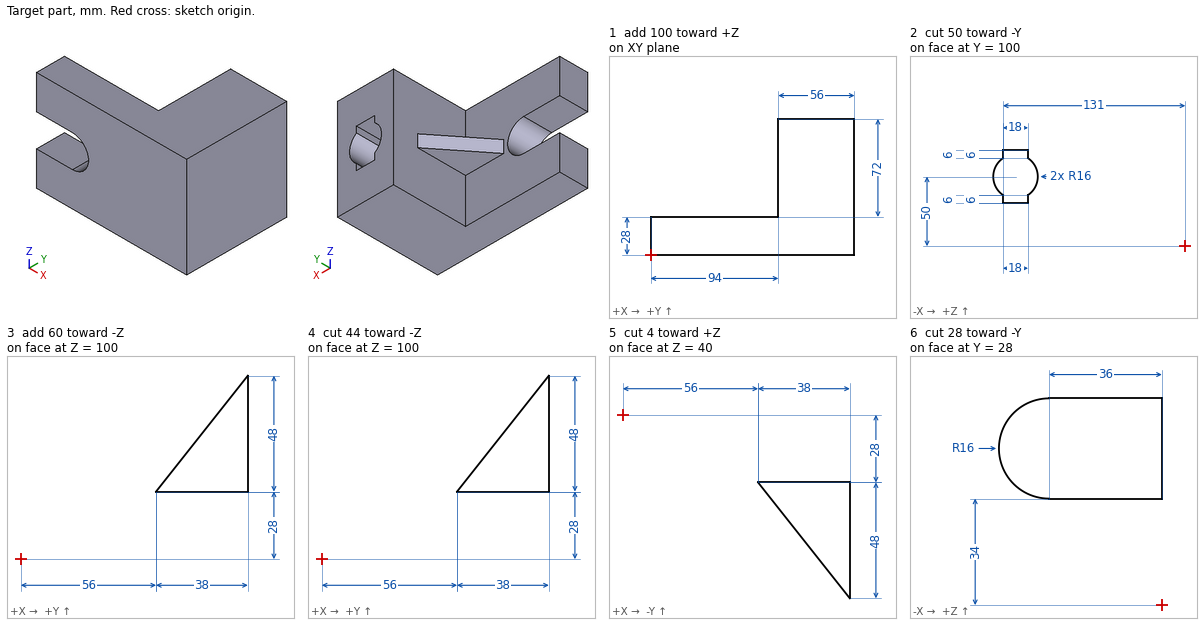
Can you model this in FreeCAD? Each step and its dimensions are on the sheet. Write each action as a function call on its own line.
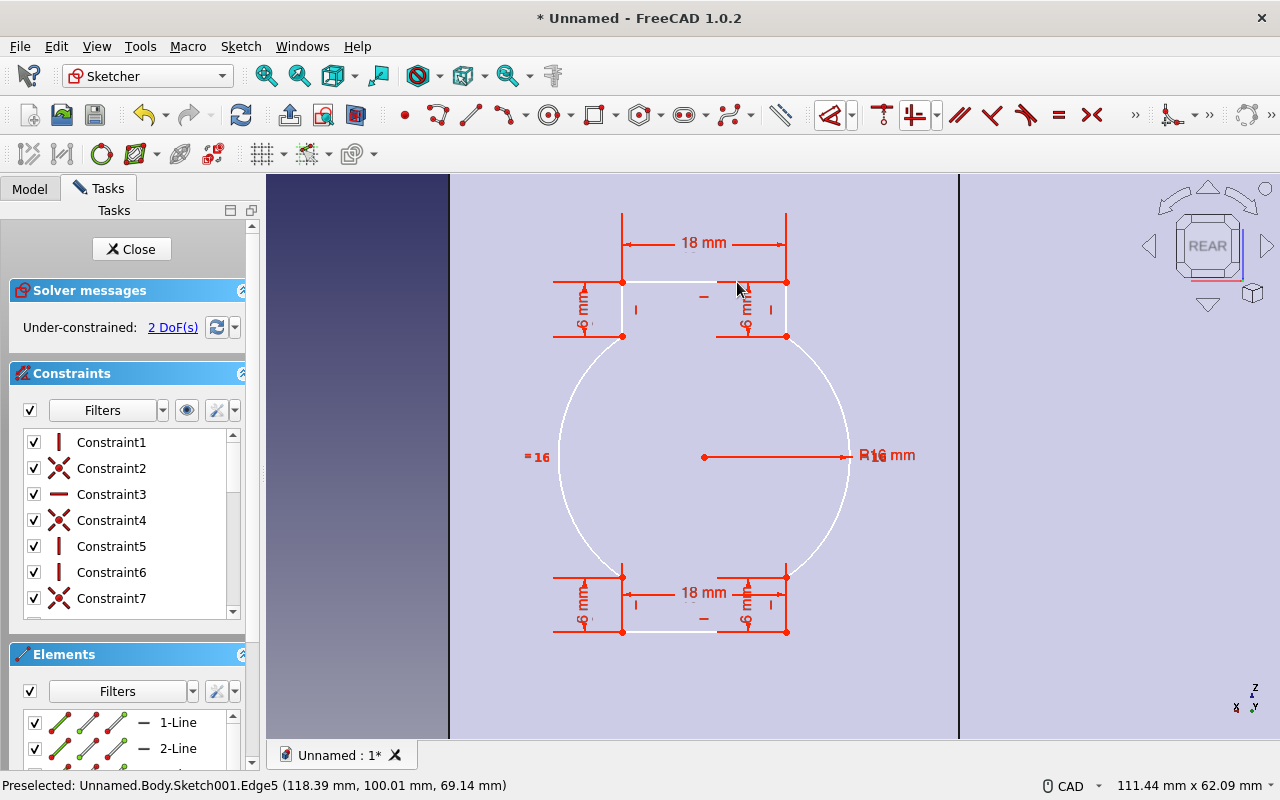
click(704, 457)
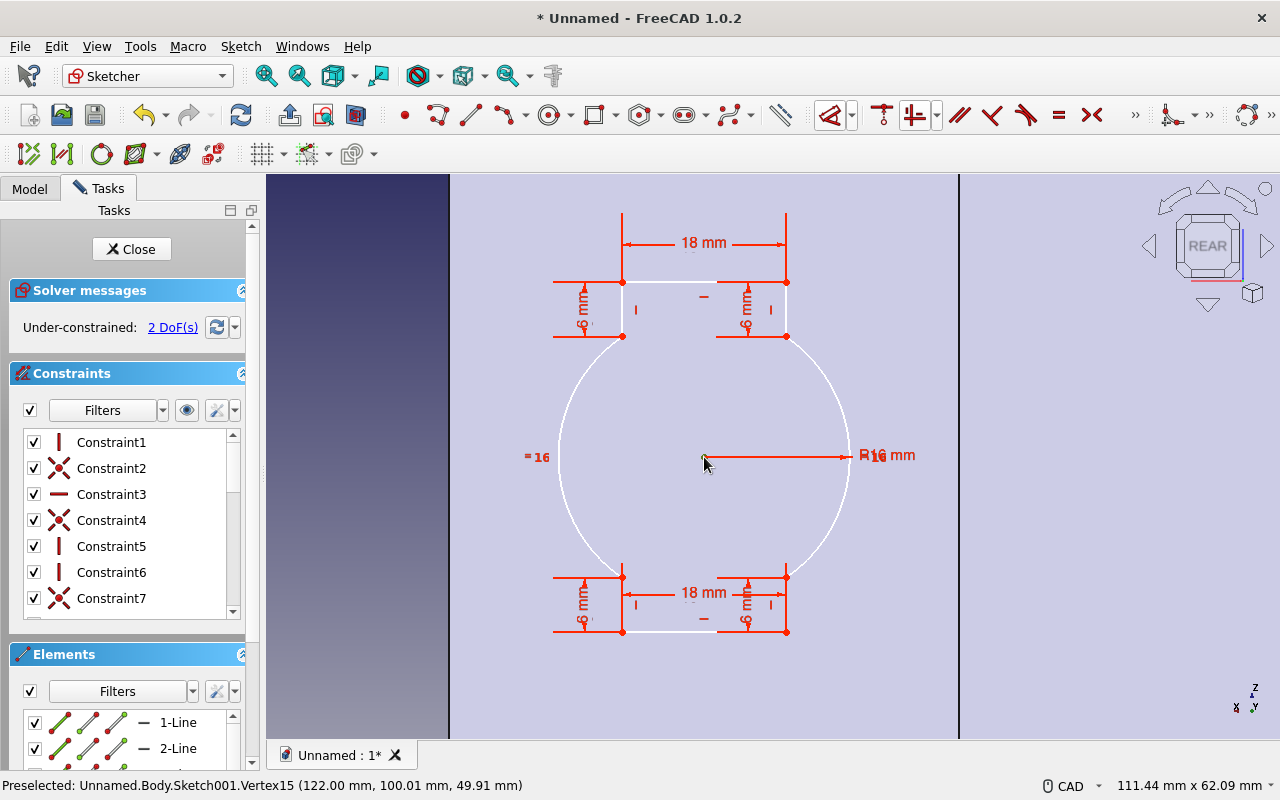
click(852, 116)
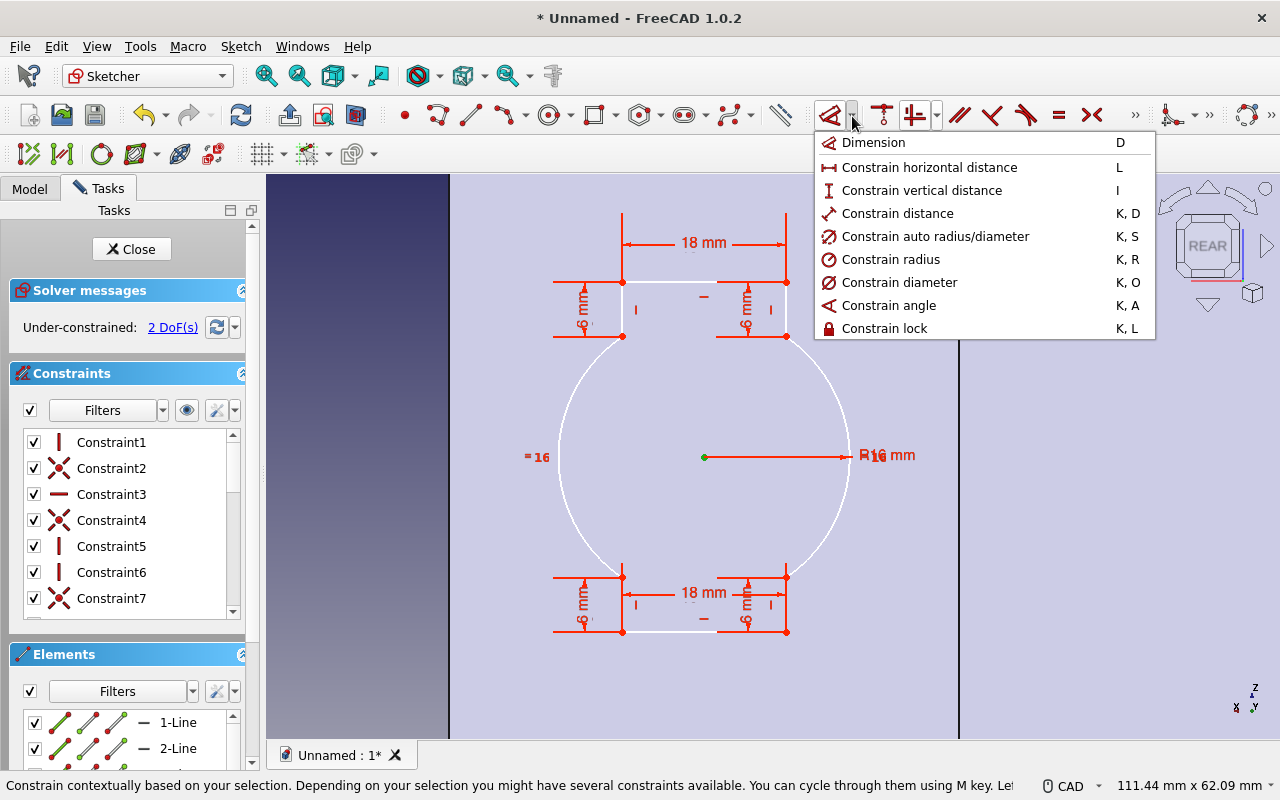
click(985, 190)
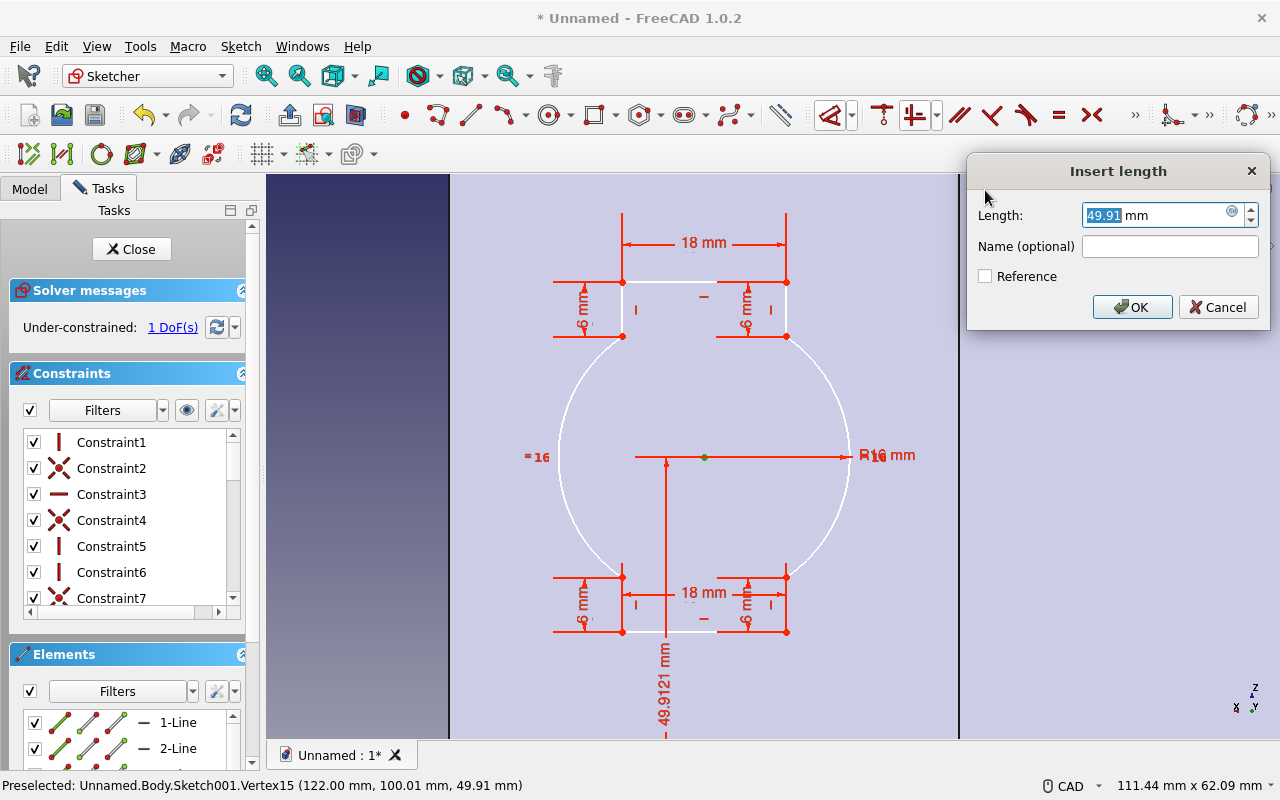
text(50)
key(Return)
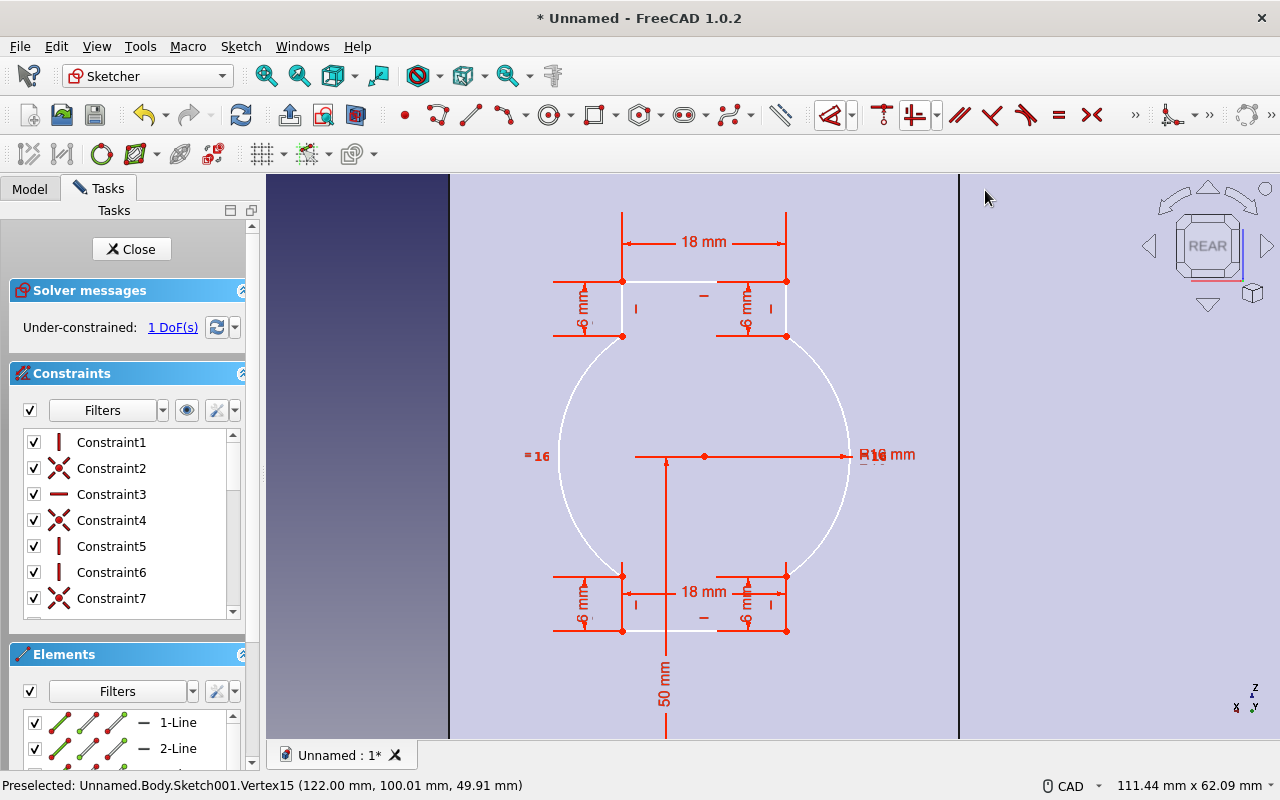
click(622, 577)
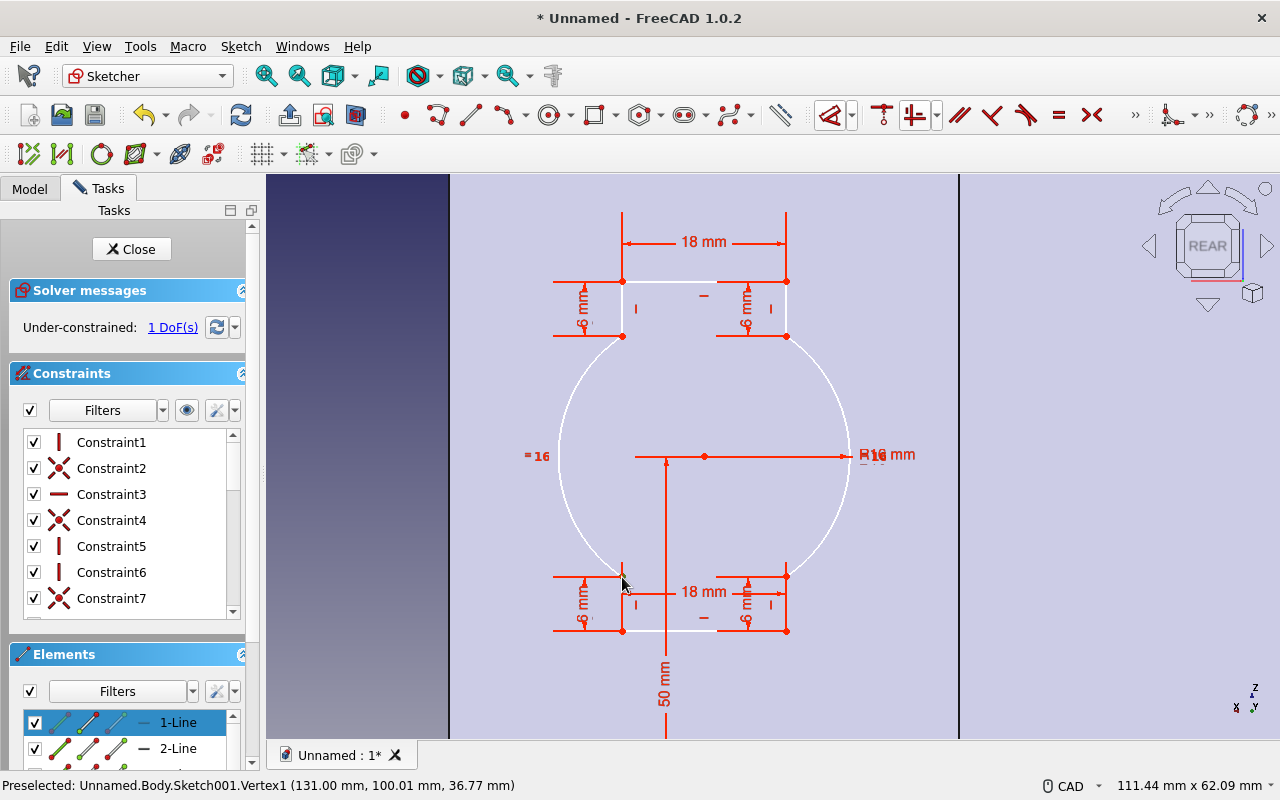
click(852, 116)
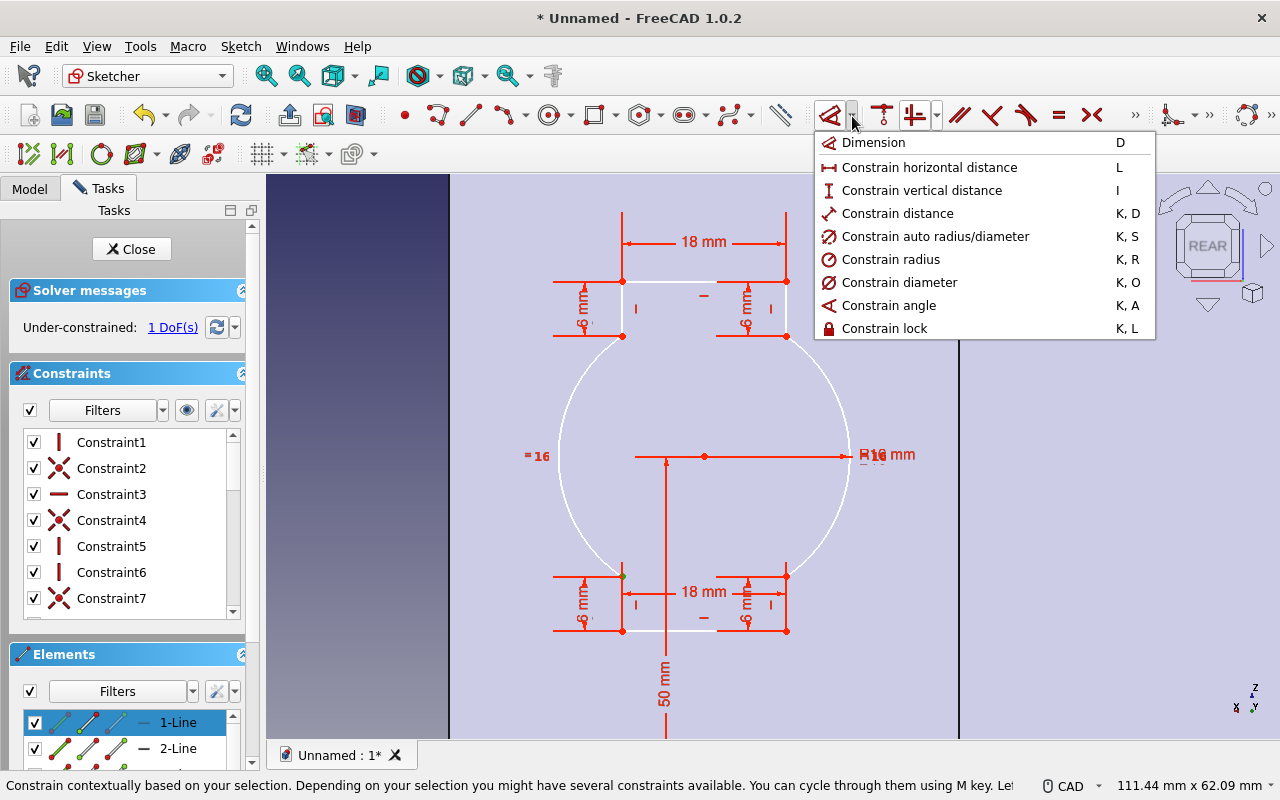
click(985, 168)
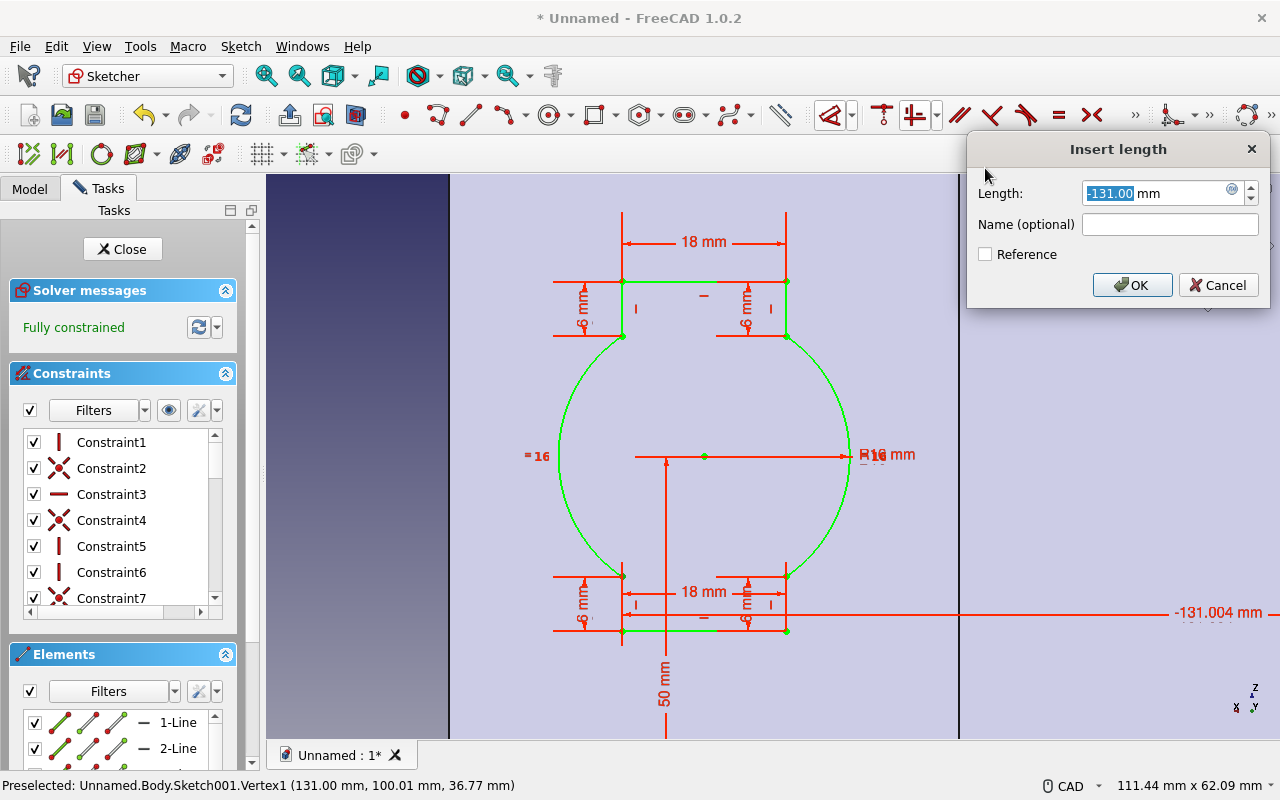
text(-131)
key(Return)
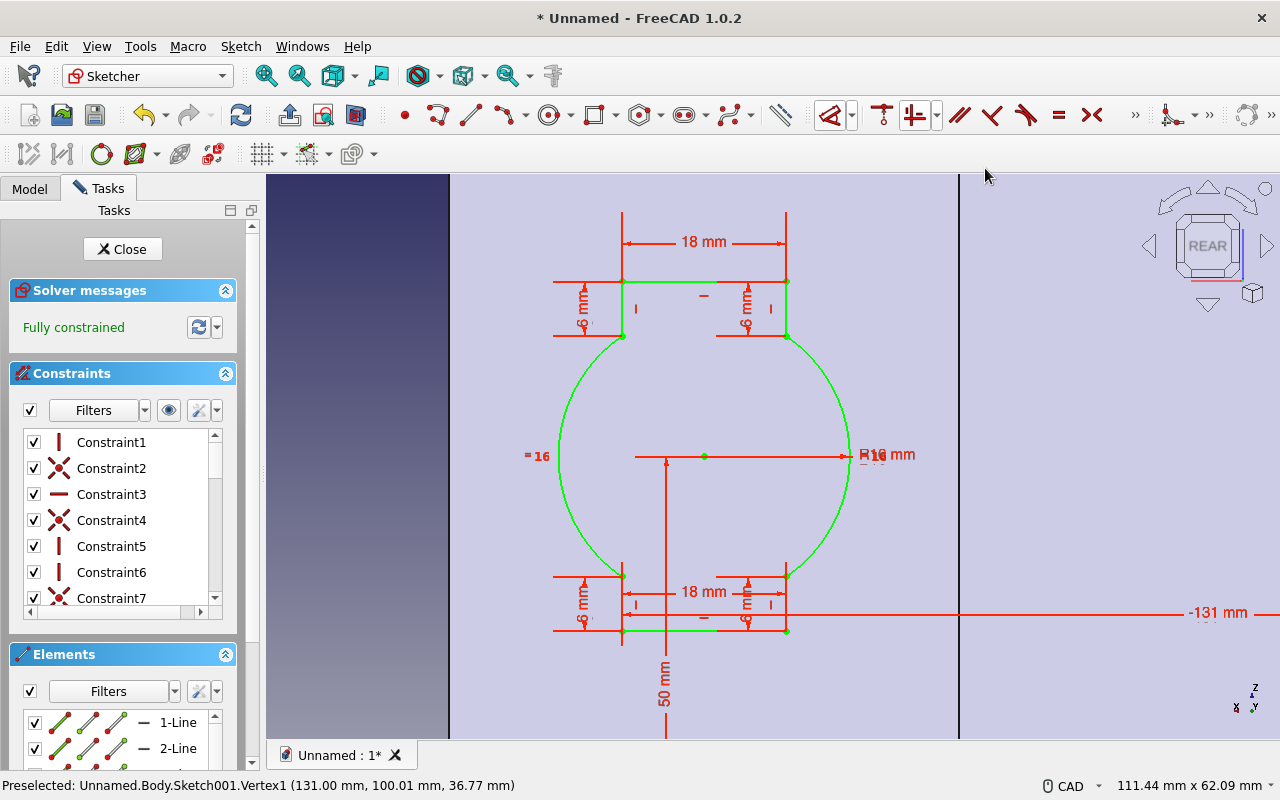
click(123, 249)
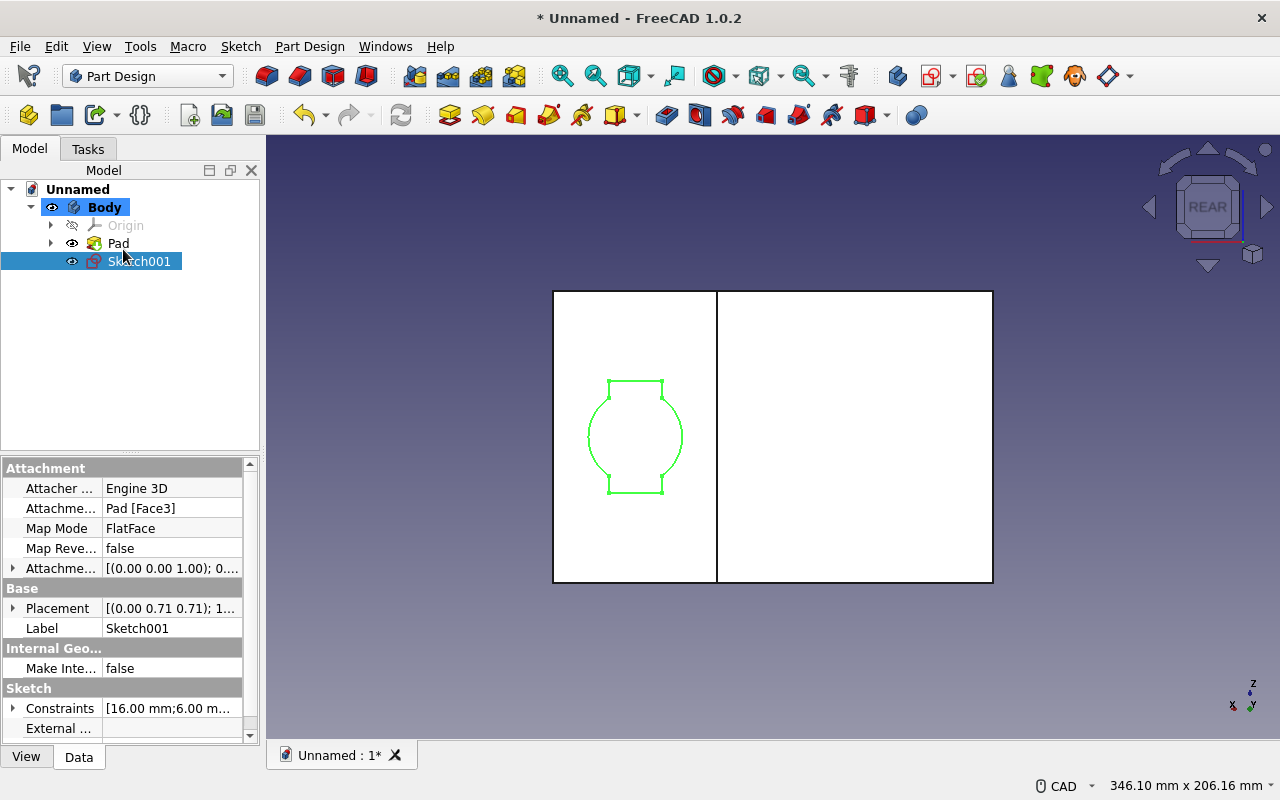
click(667, 116)